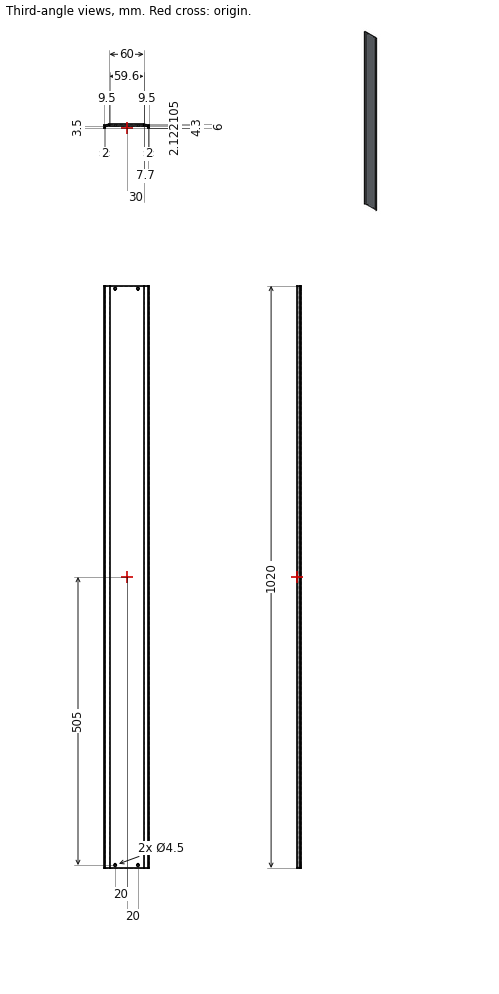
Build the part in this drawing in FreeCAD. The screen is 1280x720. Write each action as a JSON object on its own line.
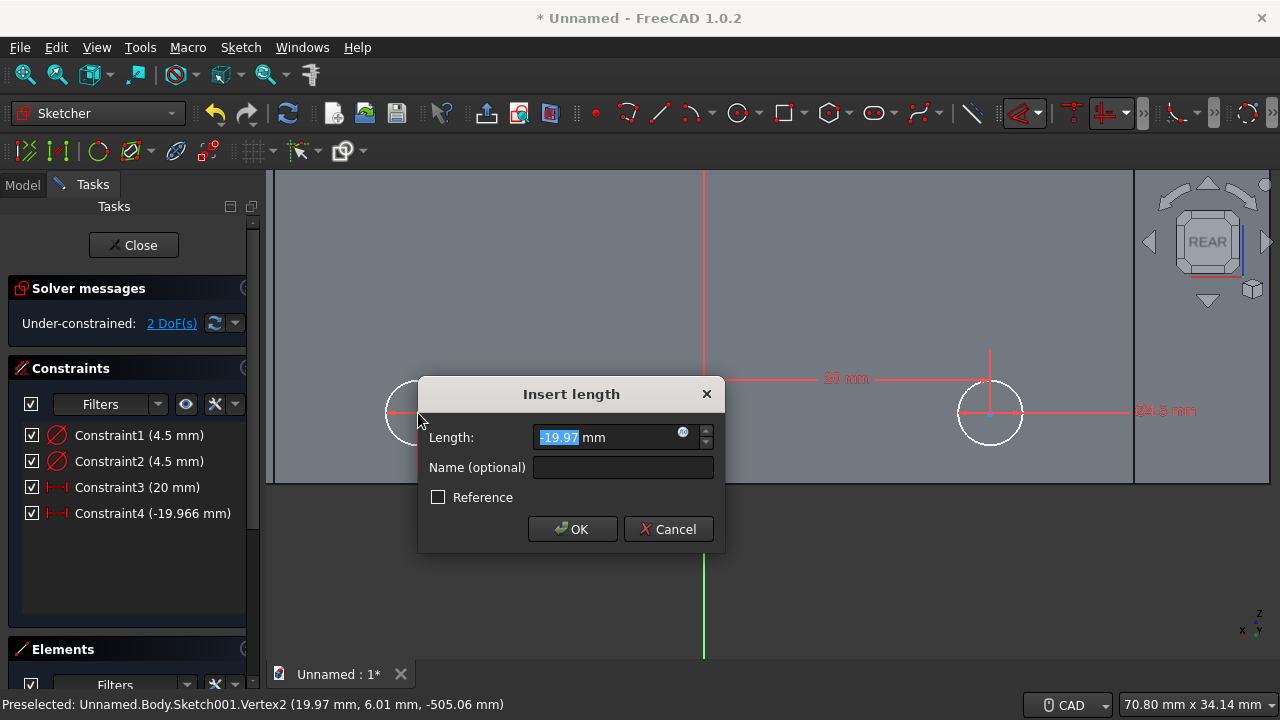
{"action": "type", "text": "-20"}
{"action": "key", "text": "Return"}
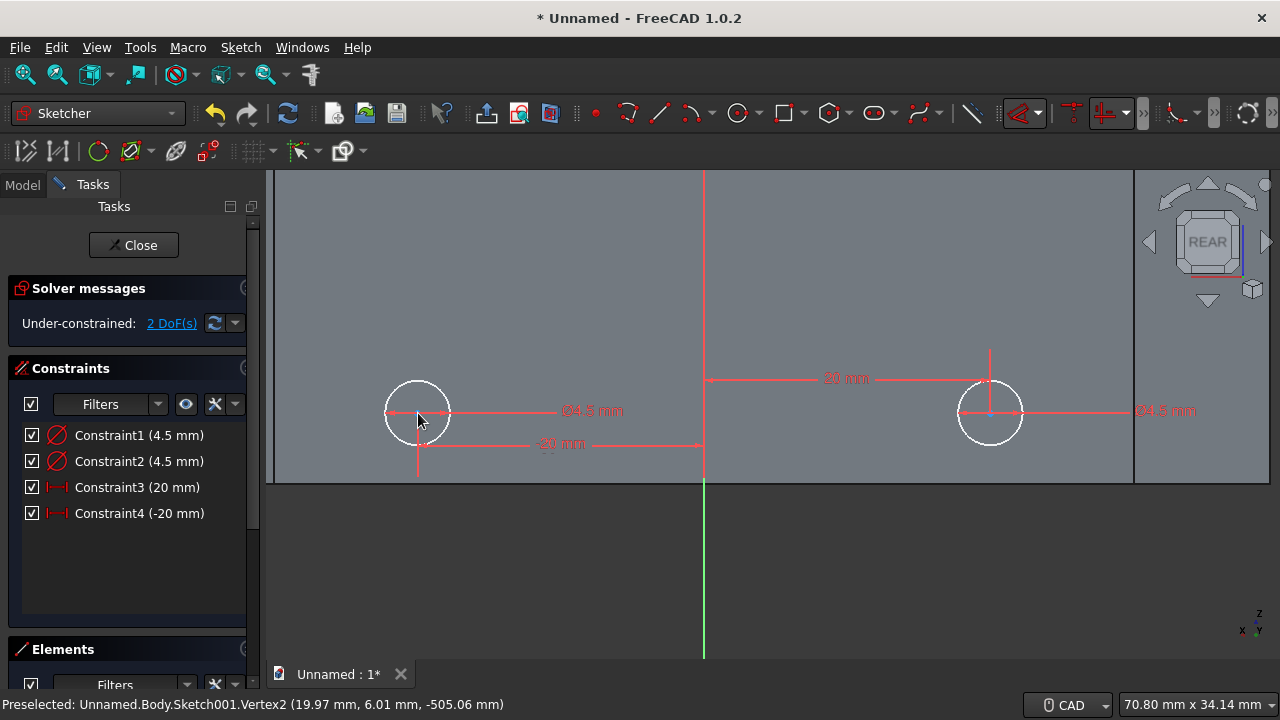
{"action": "left_click", "coordinate": [990, 413]}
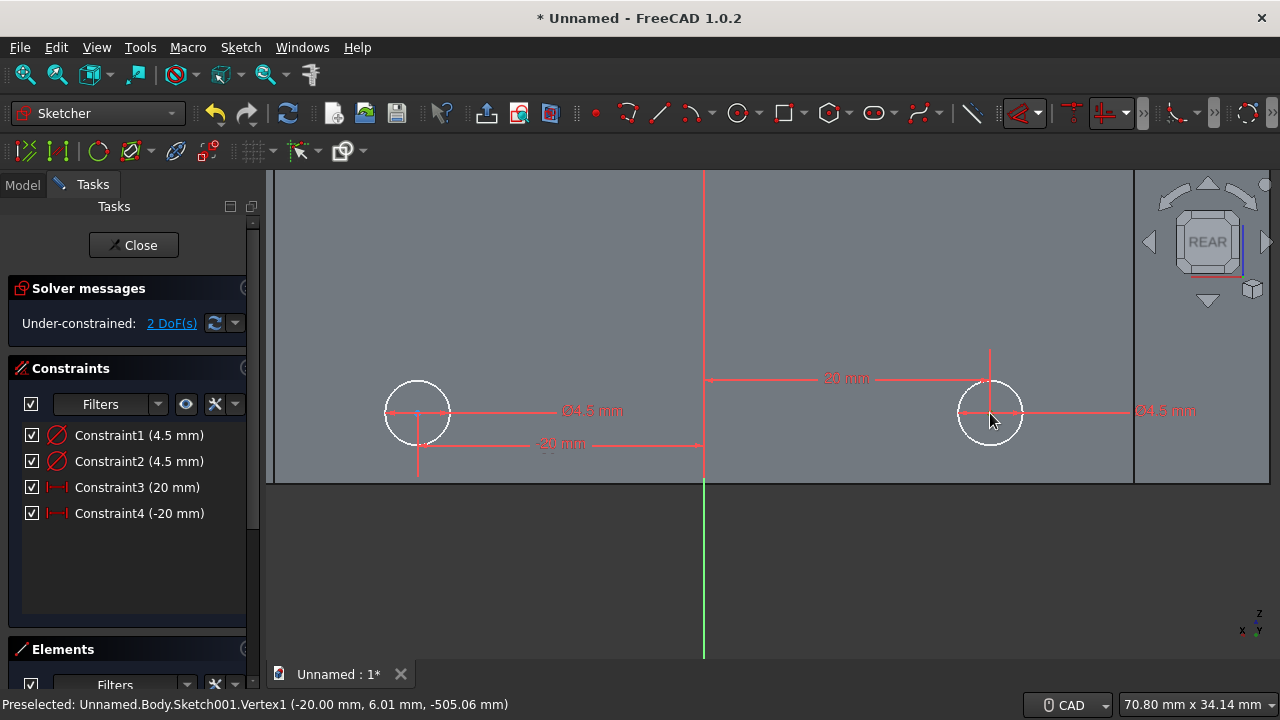
{"action": "key", "text": "i"}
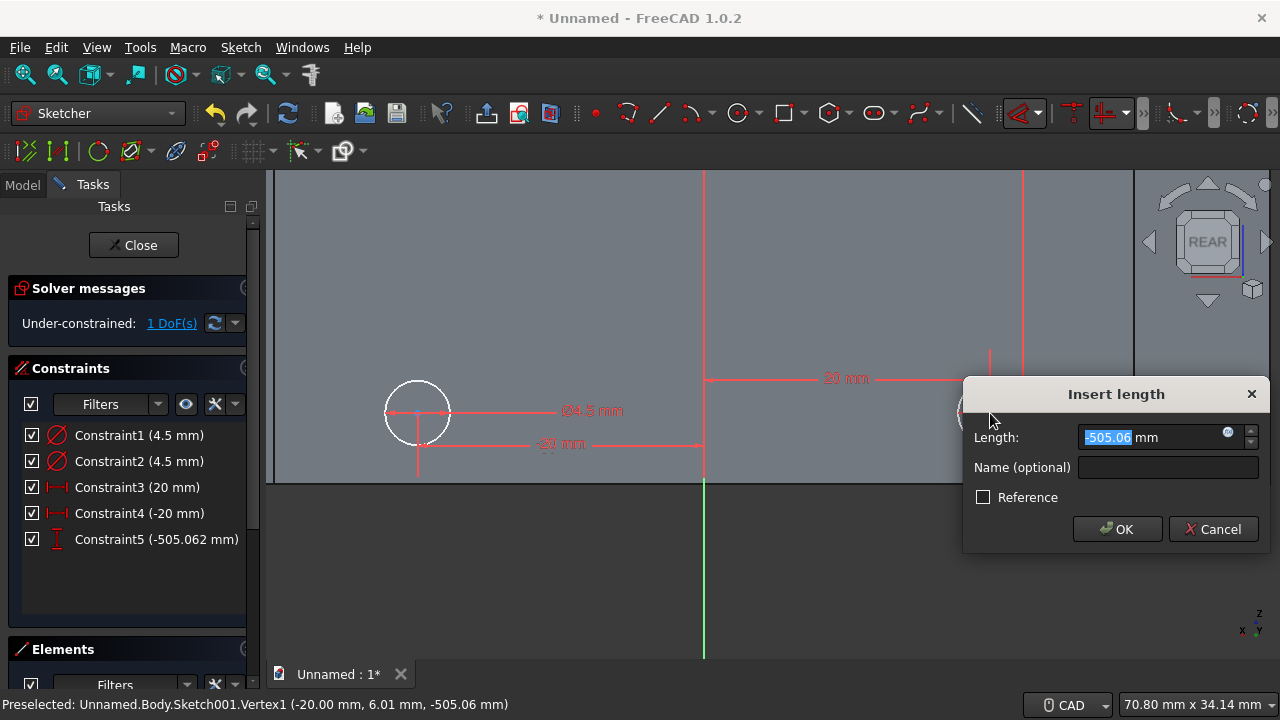
{"action": "type", "text": "-505"}
{"action": "key", "text": "Return"}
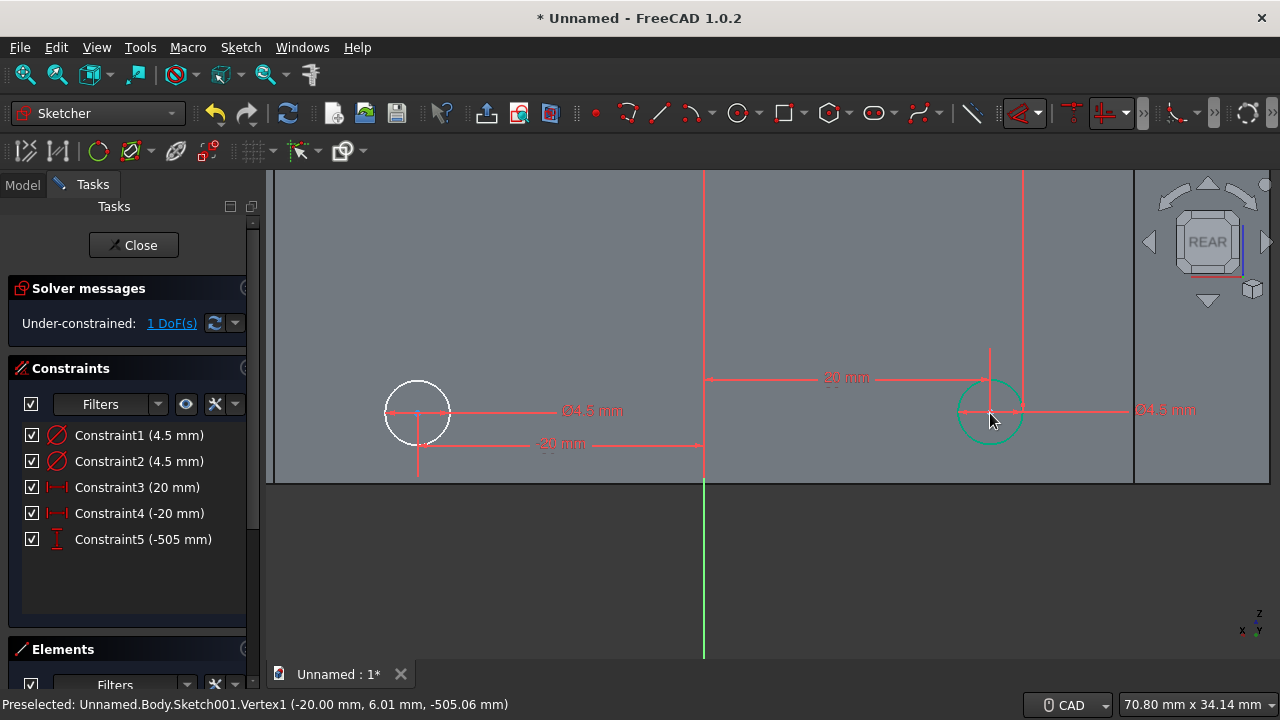
{"action": "left_click", "coordinate": [418, 413]}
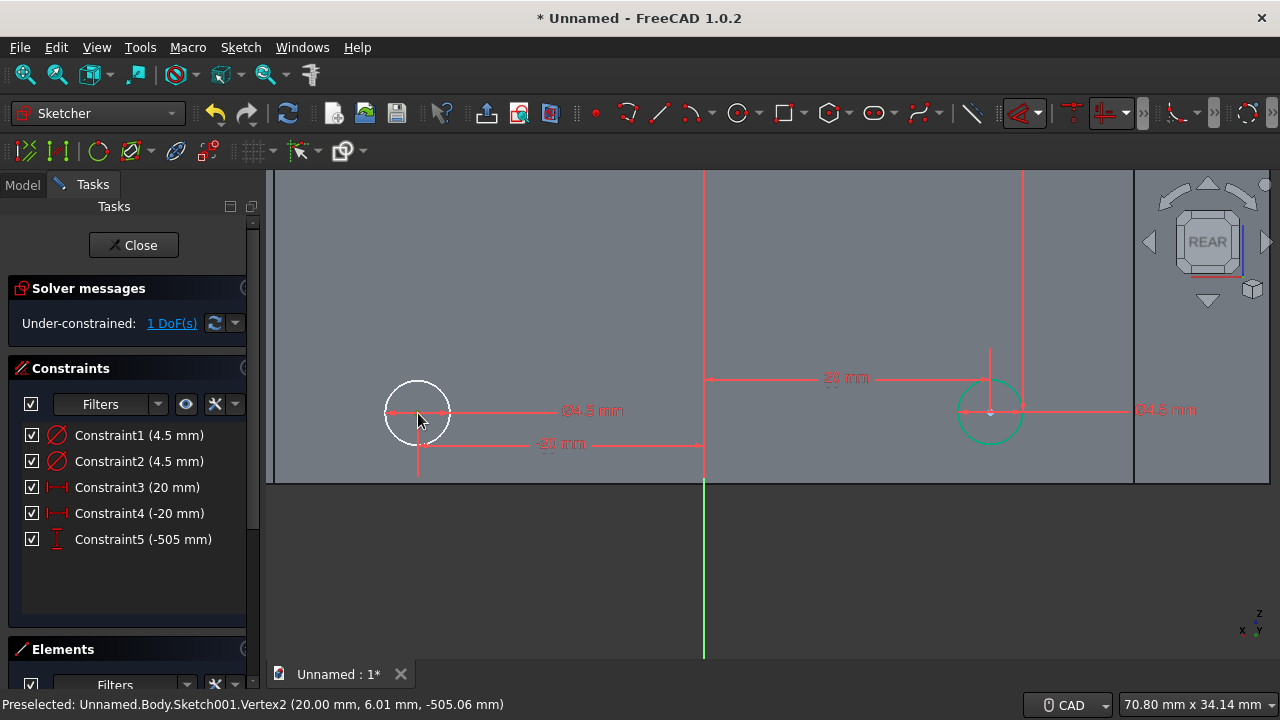
{"action": "key", "text": "i"}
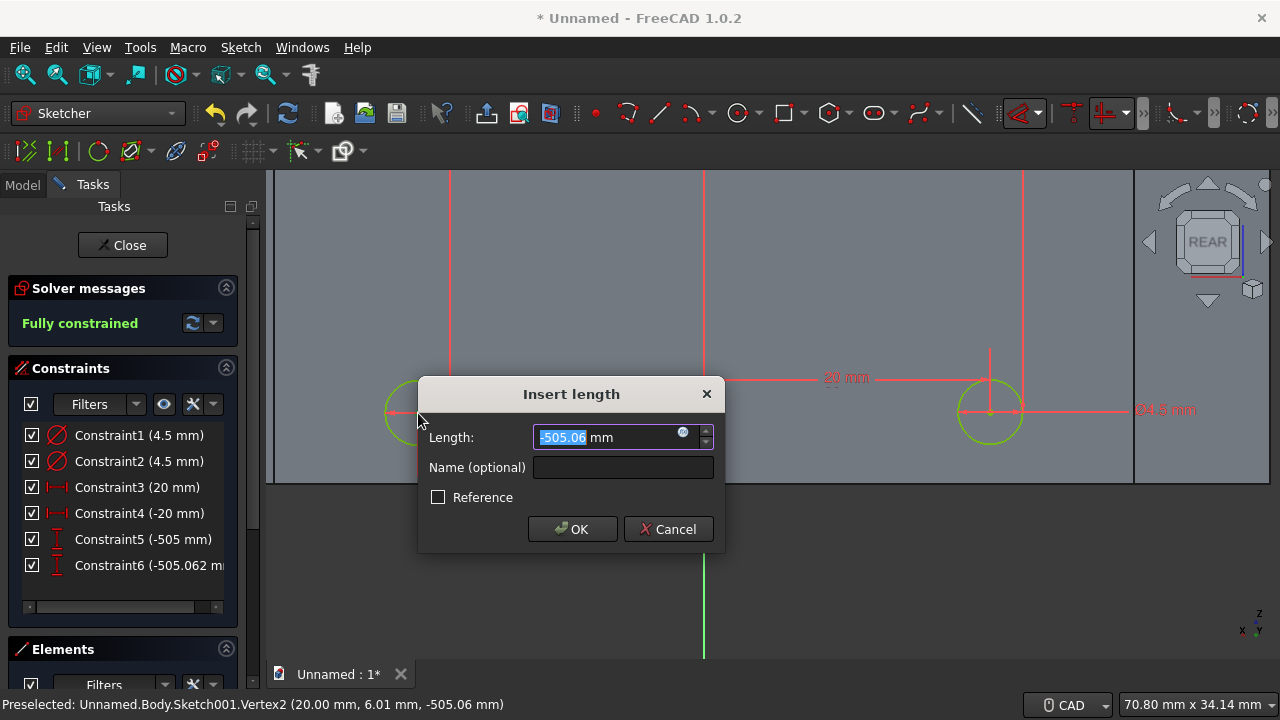
{"action": "type", "text": "-505"}
{"action": "key", "text": "Return"}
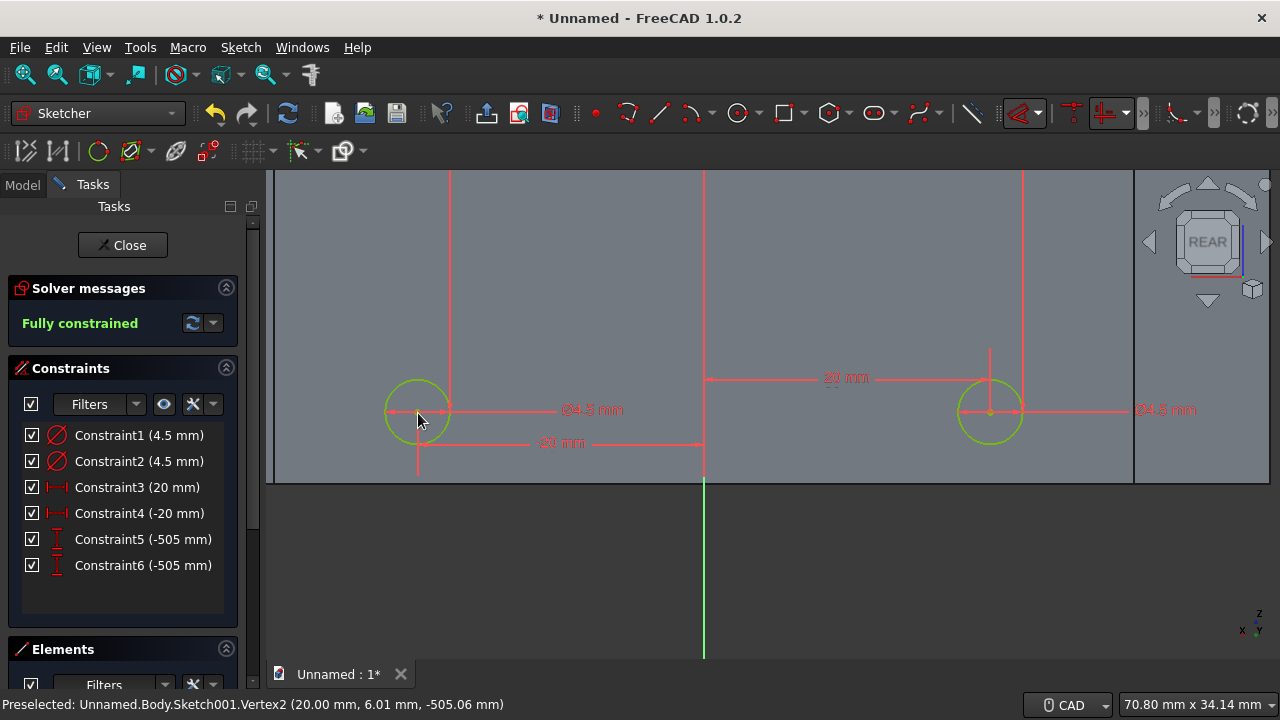
{"action": "left_click", "coordinate": [123, 245]}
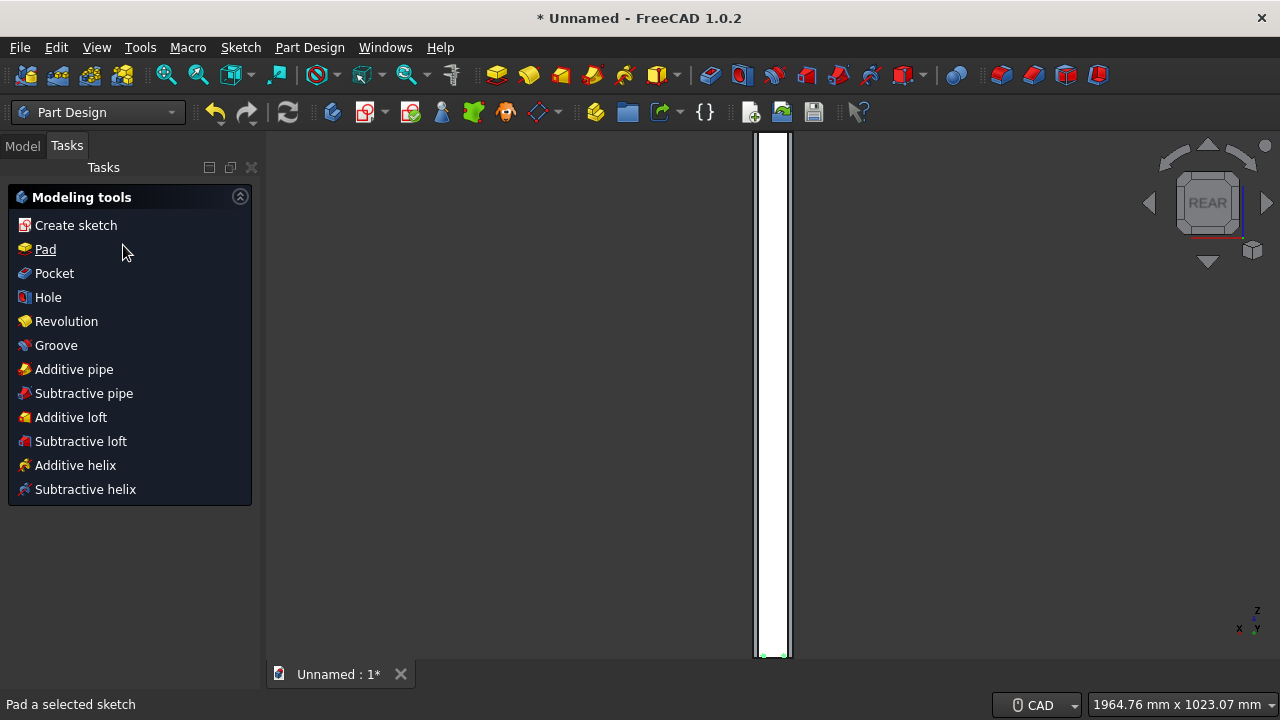
{"action": "left_click", "coordinate": [712, 76]}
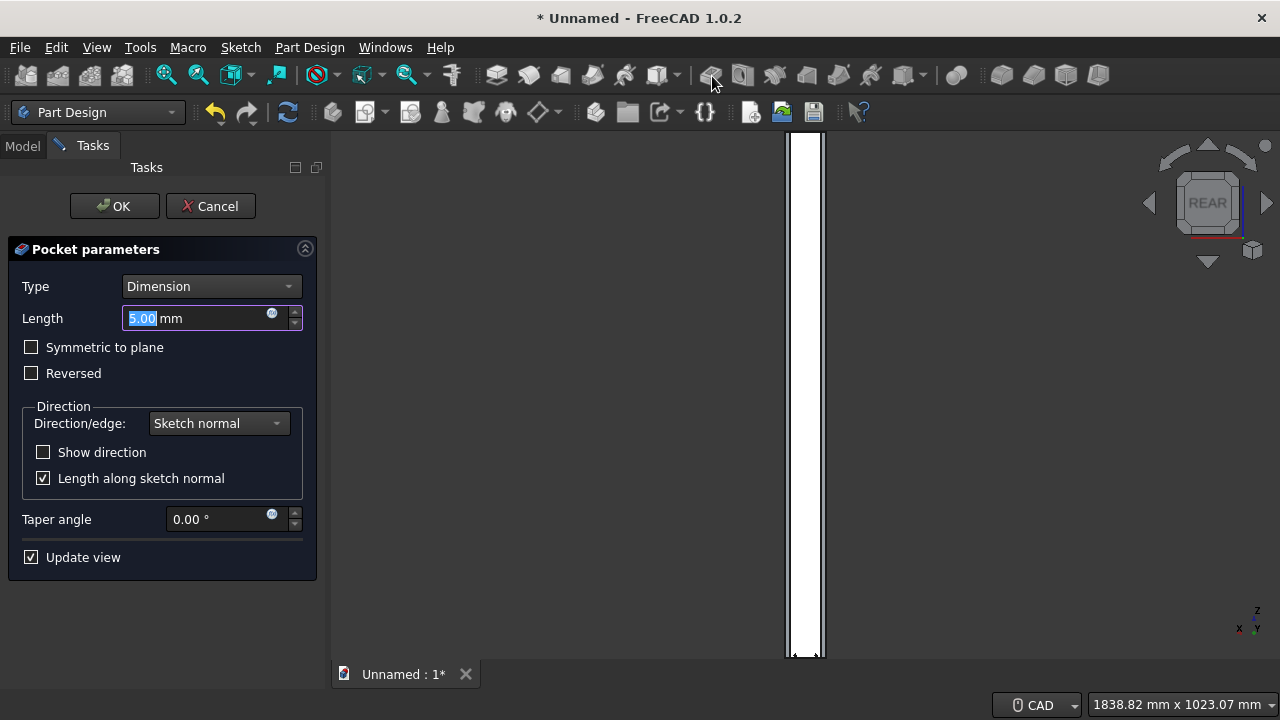
{"action": "type", "text": "20"}
{"action": "key", "text": "Tab"}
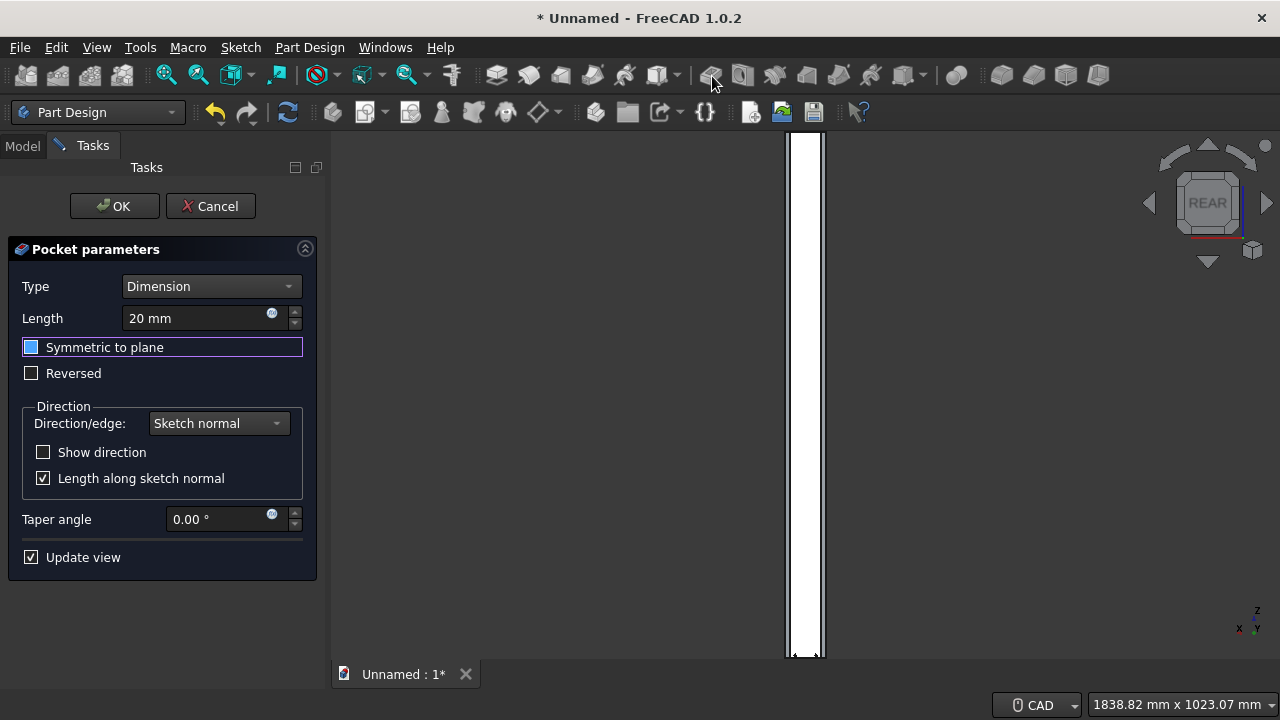
{"action": "left_click", "coordinate": [115, 206]}